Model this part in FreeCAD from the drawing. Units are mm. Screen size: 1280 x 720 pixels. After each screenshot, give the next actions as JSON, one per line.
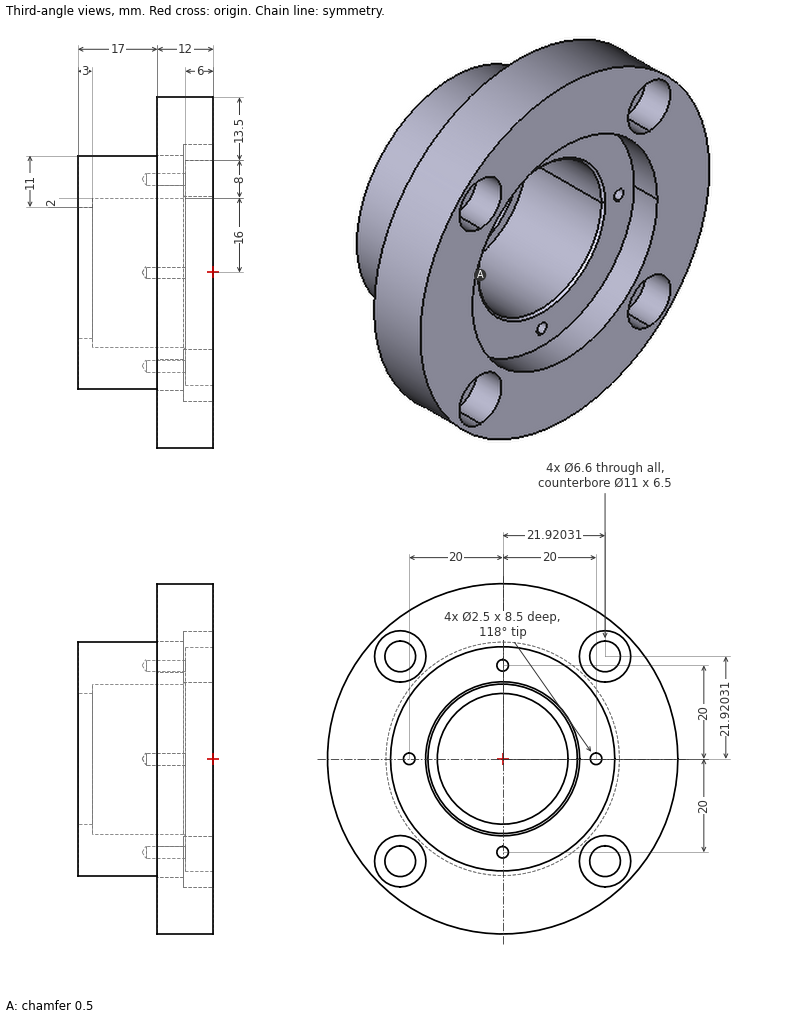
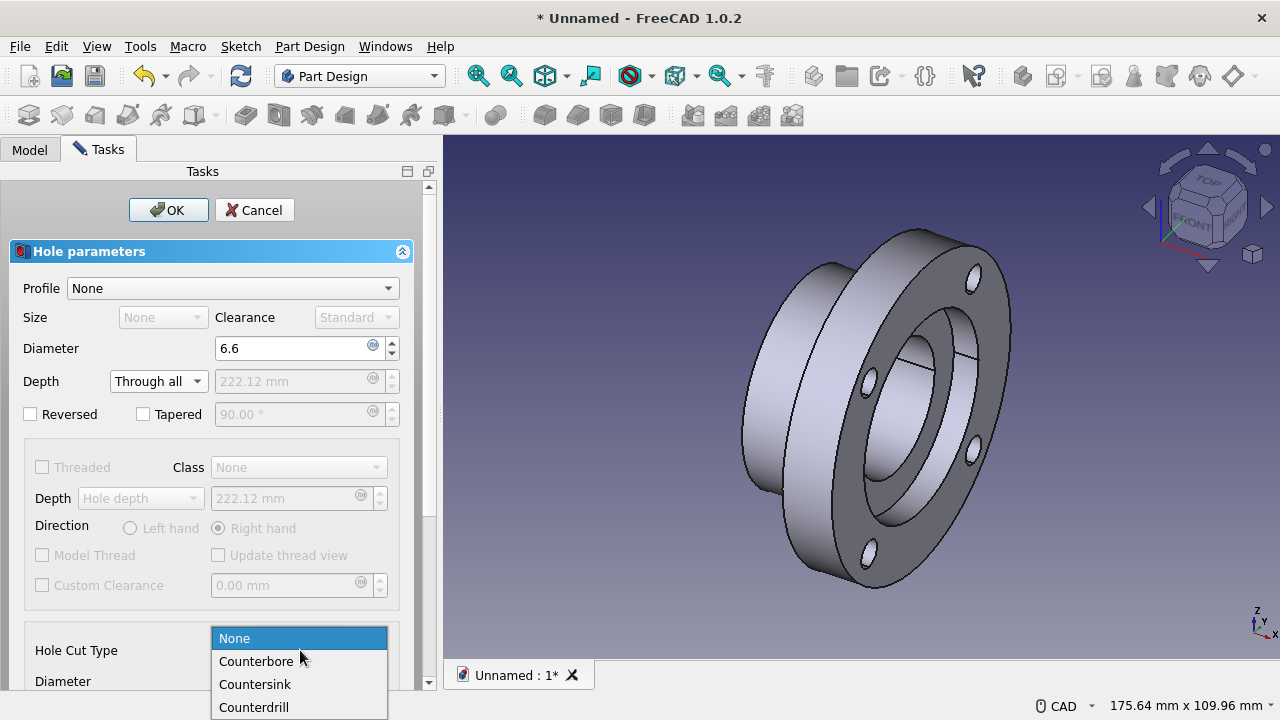
{"action": "left_click", "coordinate": [298, 662]}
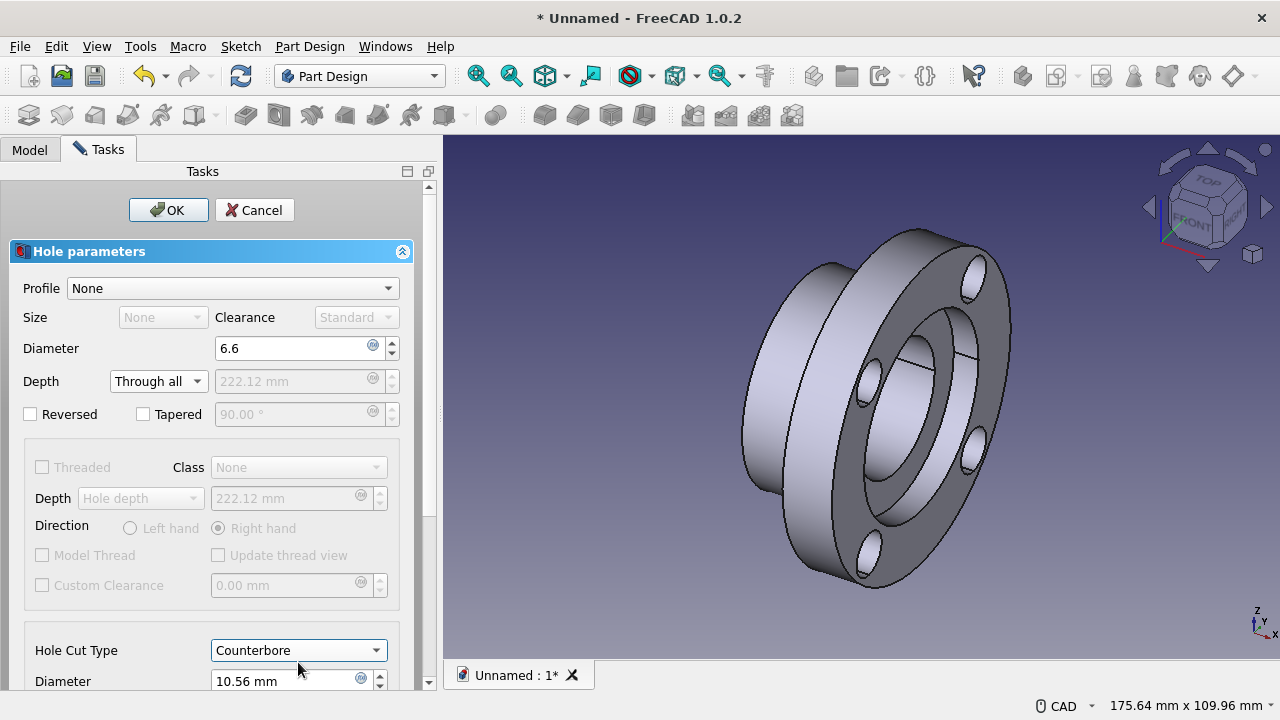
{"action": "scroll", "coordinate": [429, 436], "scroll_direction": "down", "scroll_amount": 2}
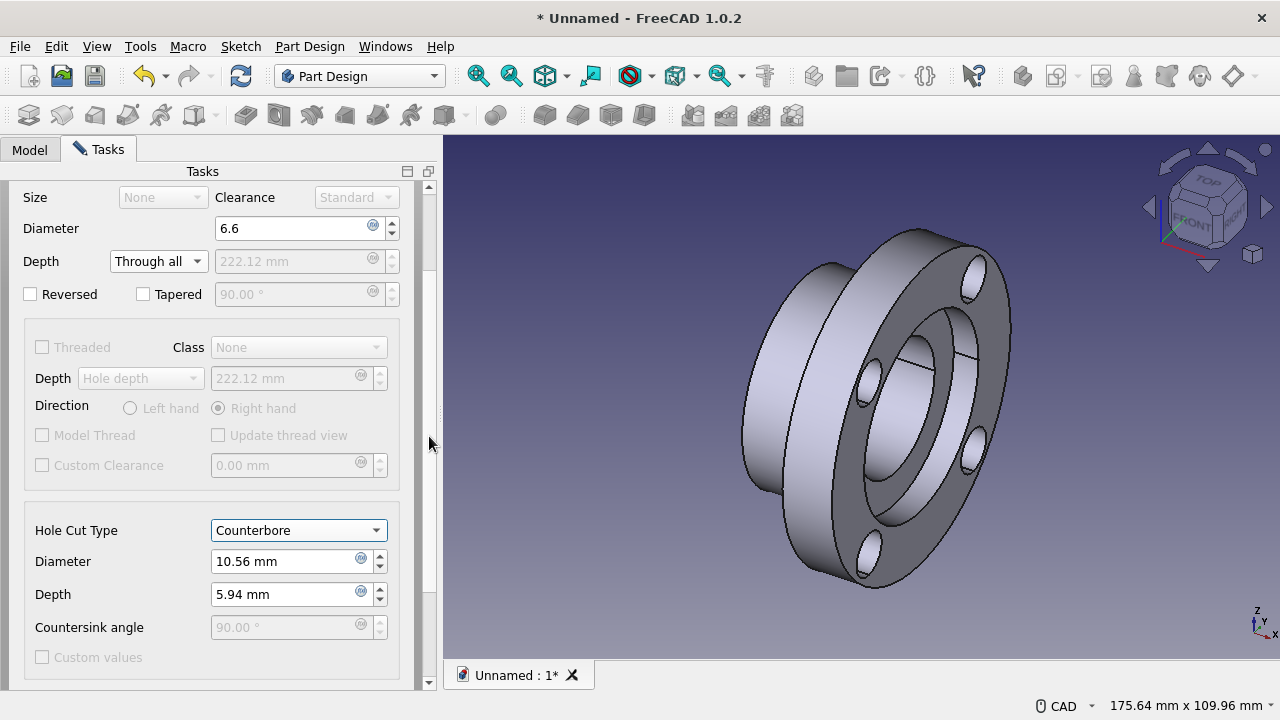
{"action": "triple_click", "coordinate": [292, 562]}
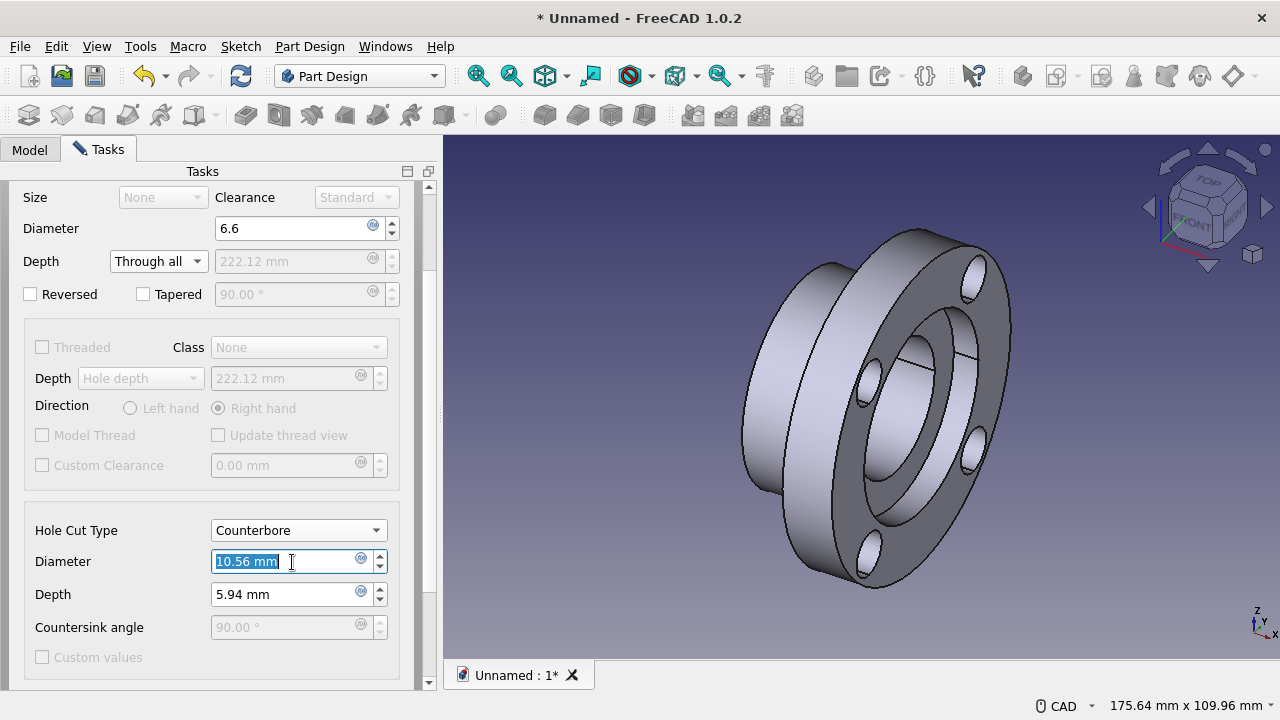
{"action": "type", "text": "11"}
{"action": "key", "text": "Tab"}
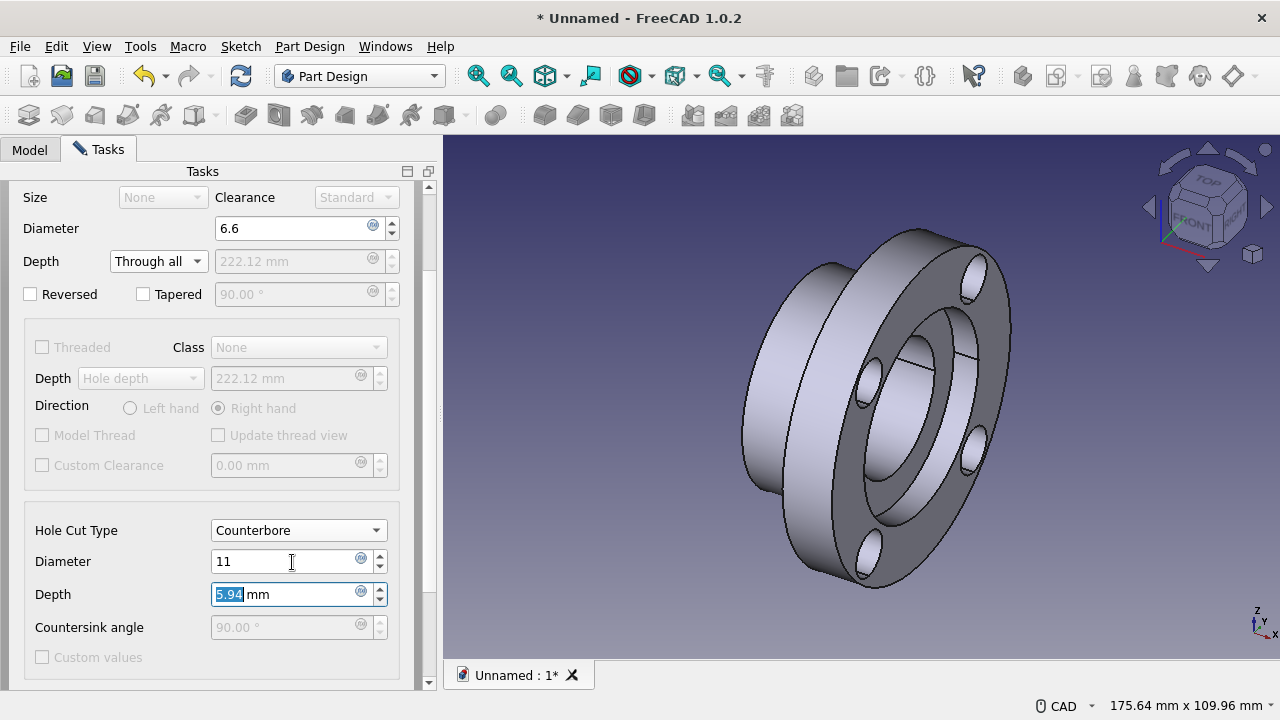
{"action": "type", "text": "6.5"}
{"action": "key", "text": "Tab"}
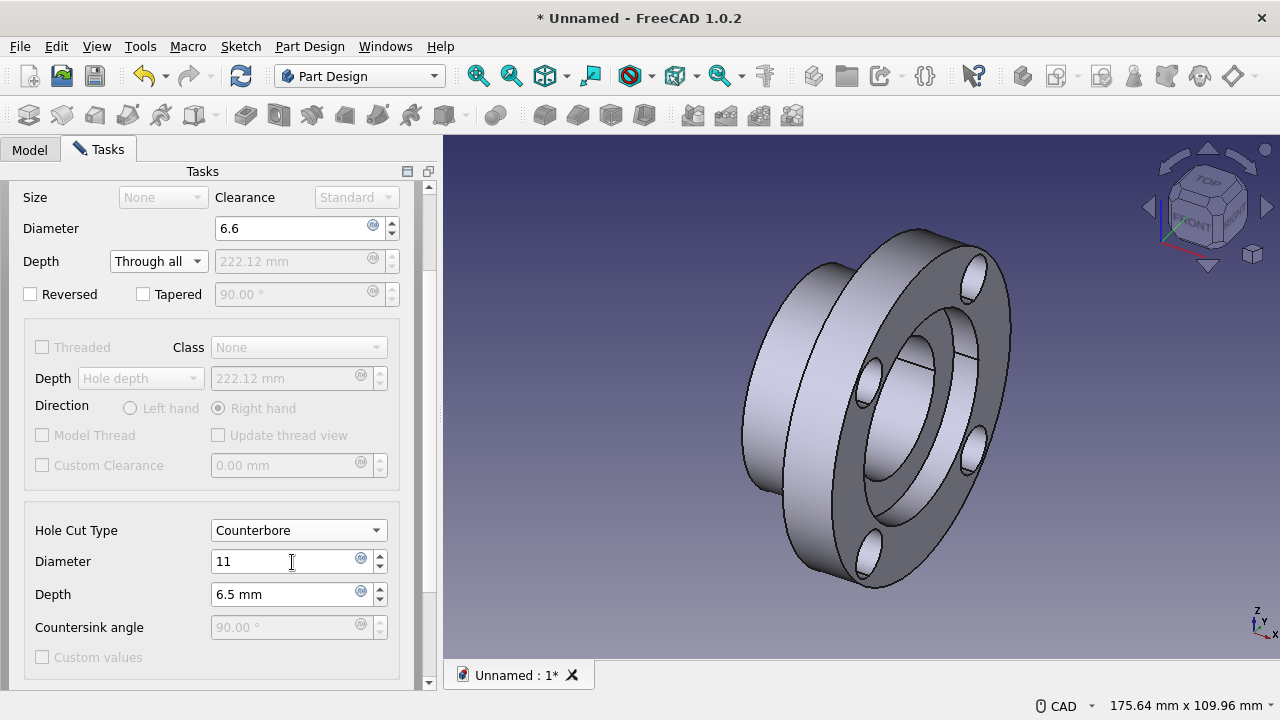
{"action": "scroll", "coordinate": [429, 436], "scroll_direction": "up", "scroll_amount": 3}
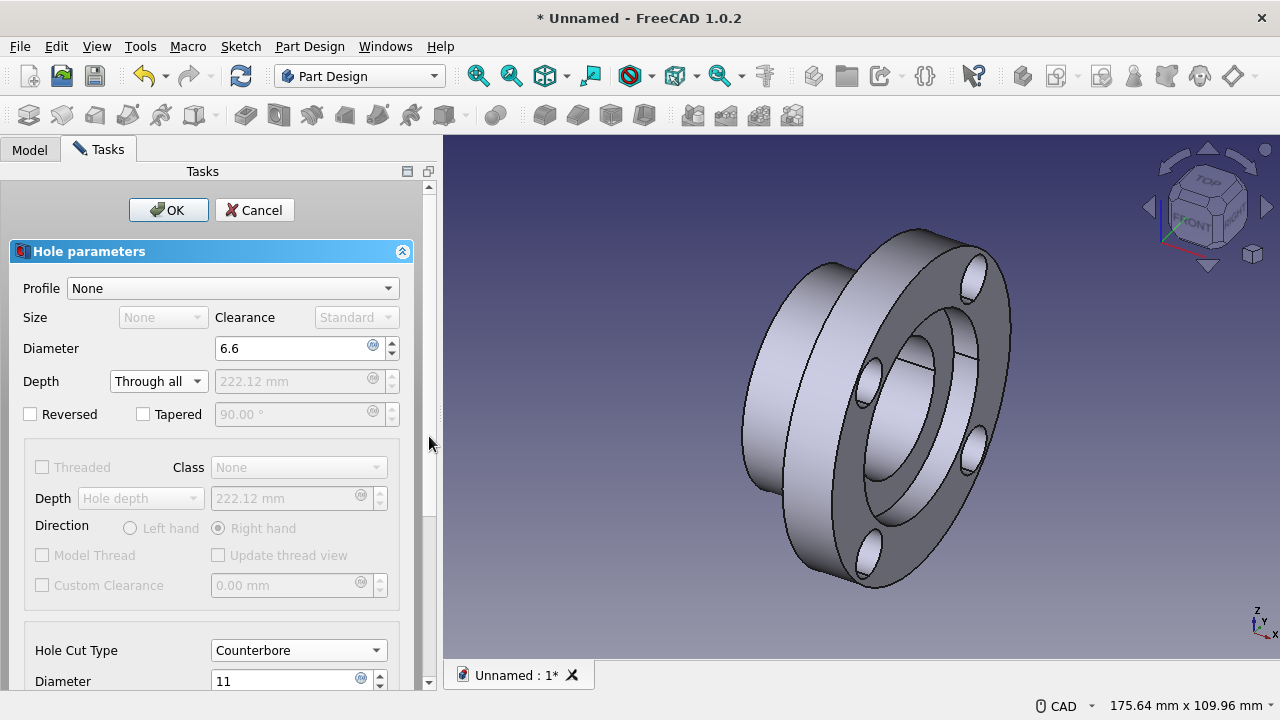
{"action": "left_click", "coordinate": [169, 210]}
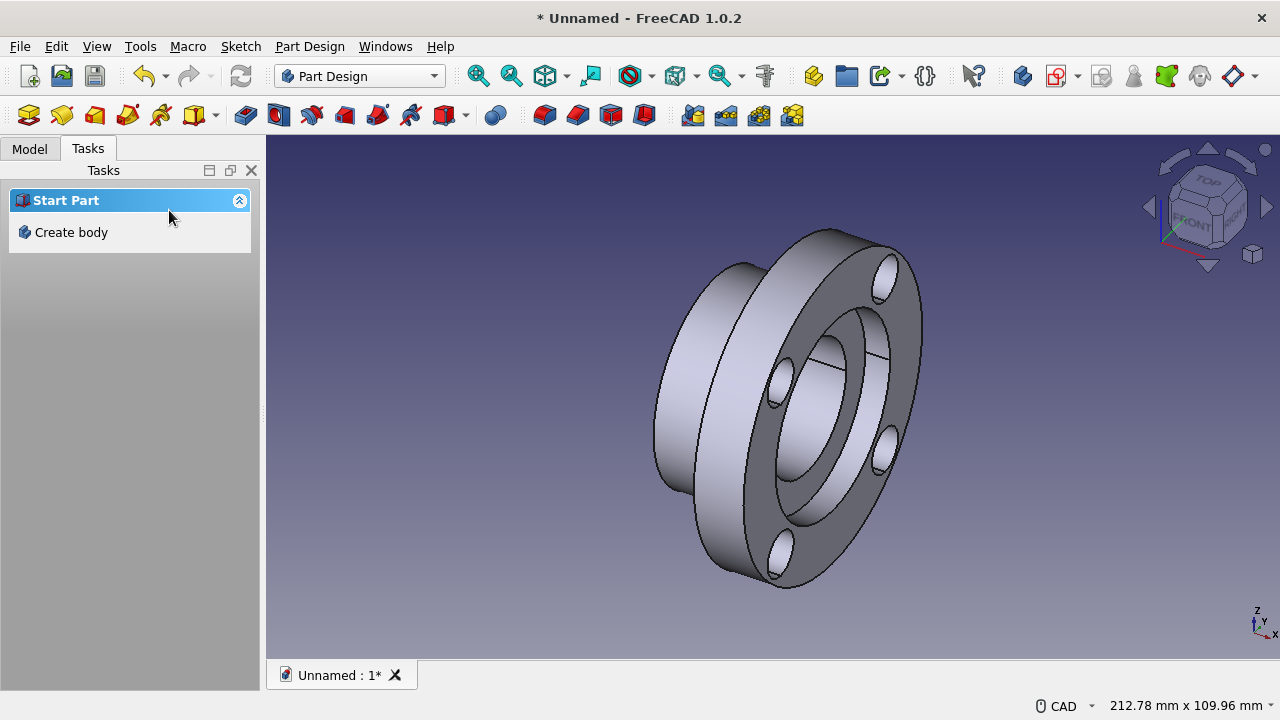
{"action": "left_click", "coordinate": [857, 359]}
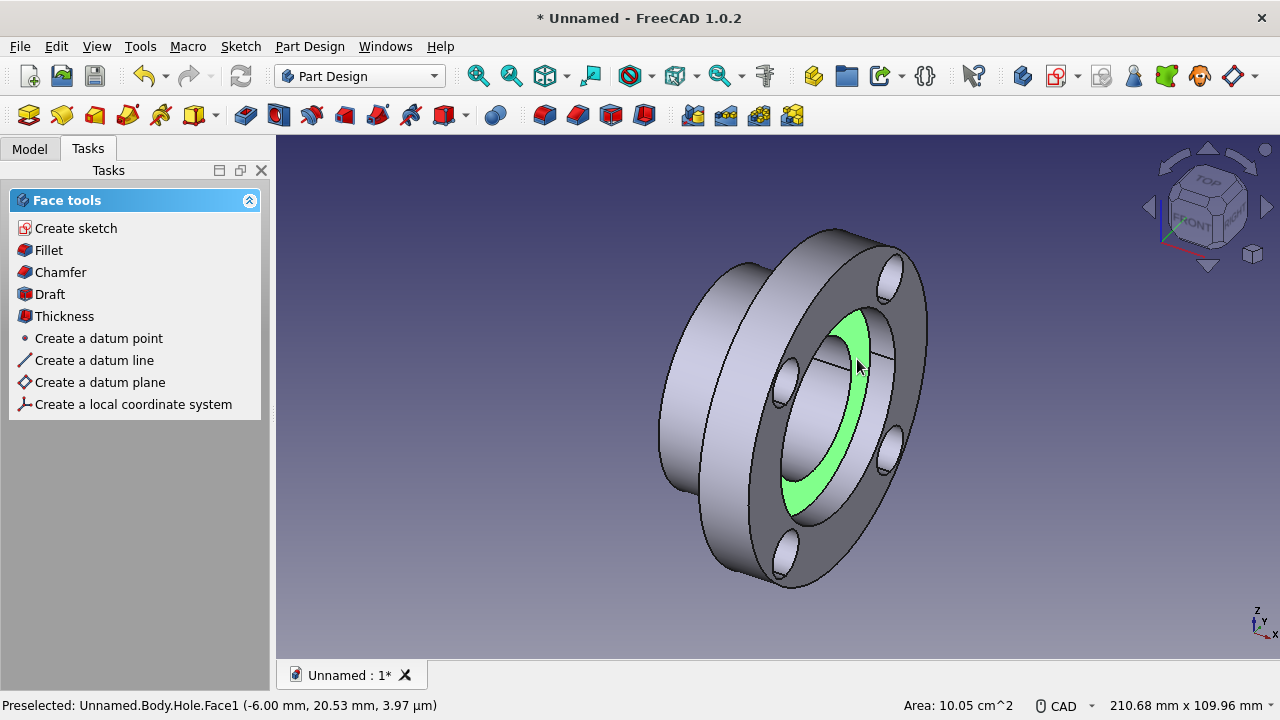
{"action": "left_click", "coordinate": [1056, 76]}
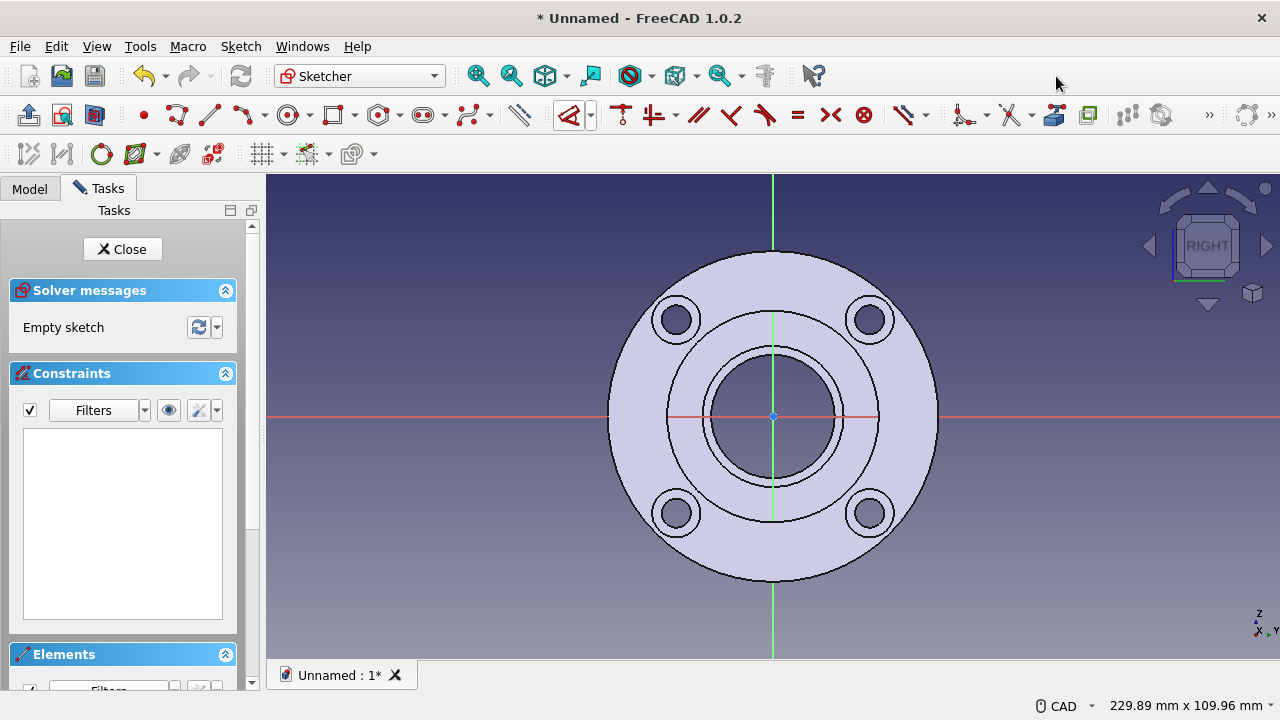
{"action": "key", "text": "q s"}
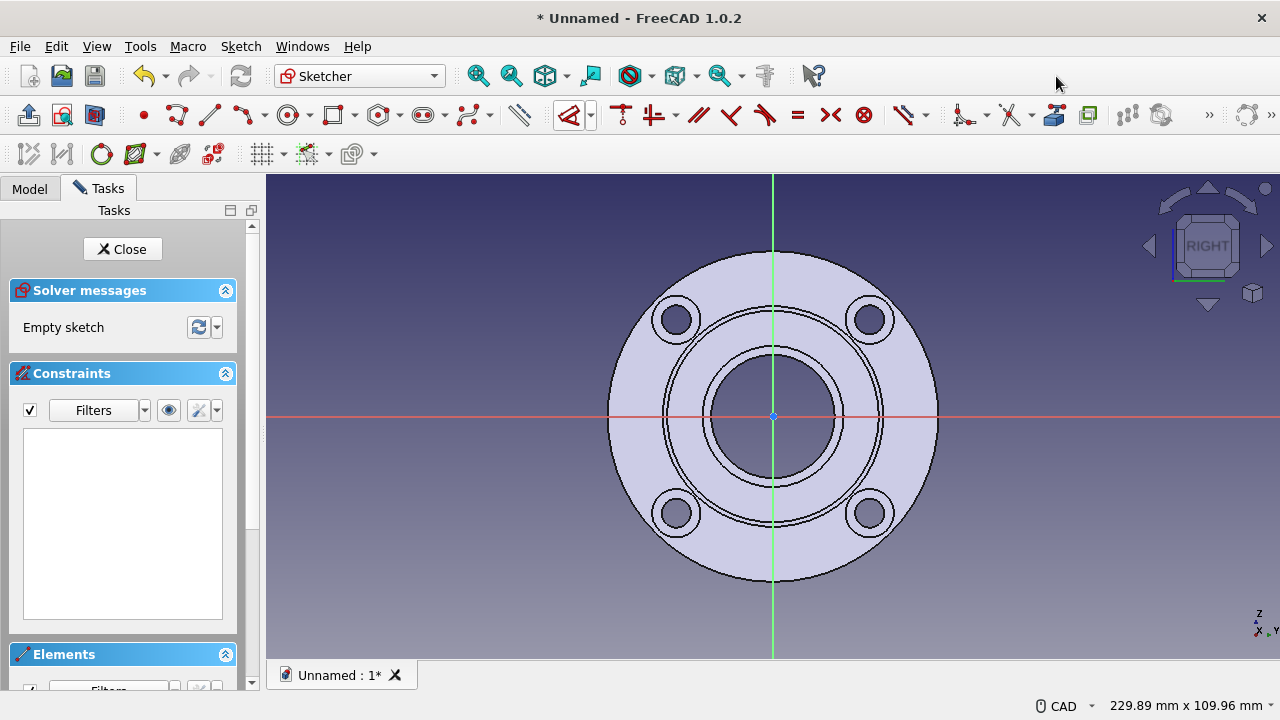
{"action": "scroll", "coordinate": [912, 416], "scroll_direction": "up", "scroll_amount": 2}